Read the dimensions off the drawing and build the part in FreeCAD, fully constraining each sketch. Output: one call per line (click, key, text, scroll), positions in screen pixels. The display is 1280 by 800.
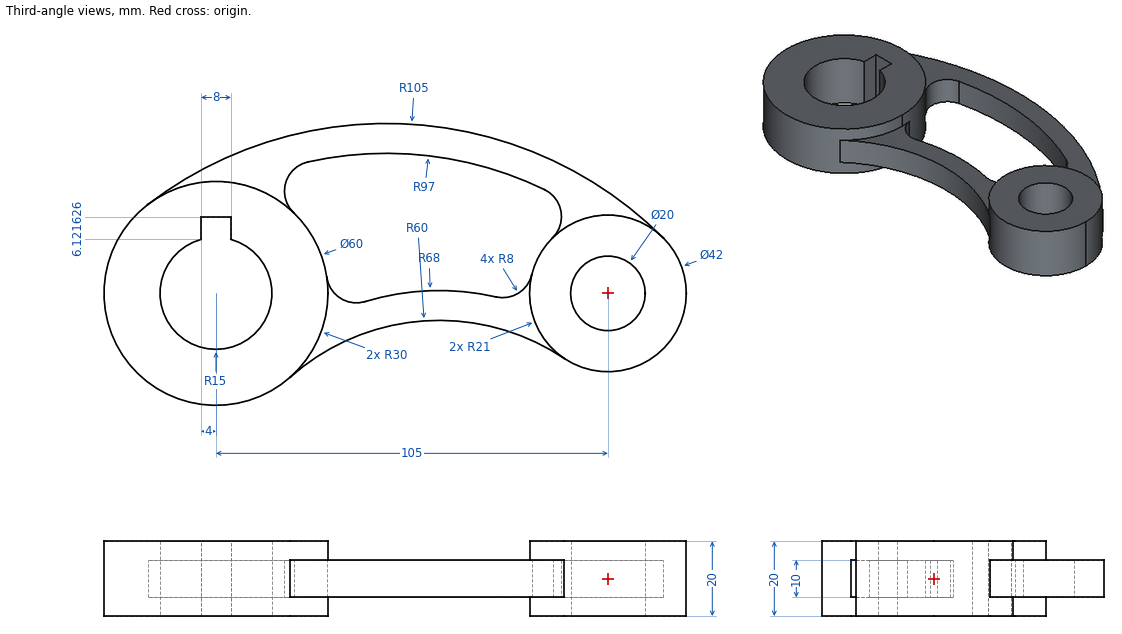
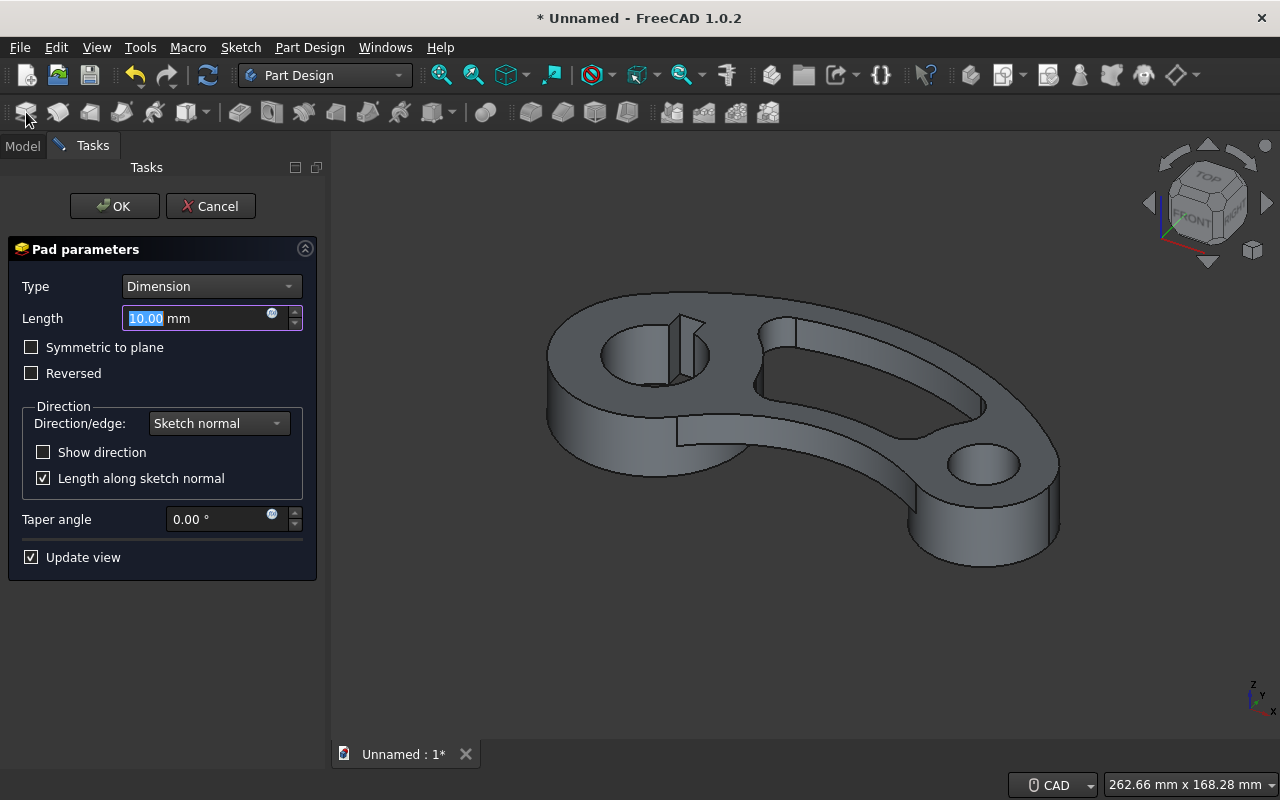
text(10)
key(Tab)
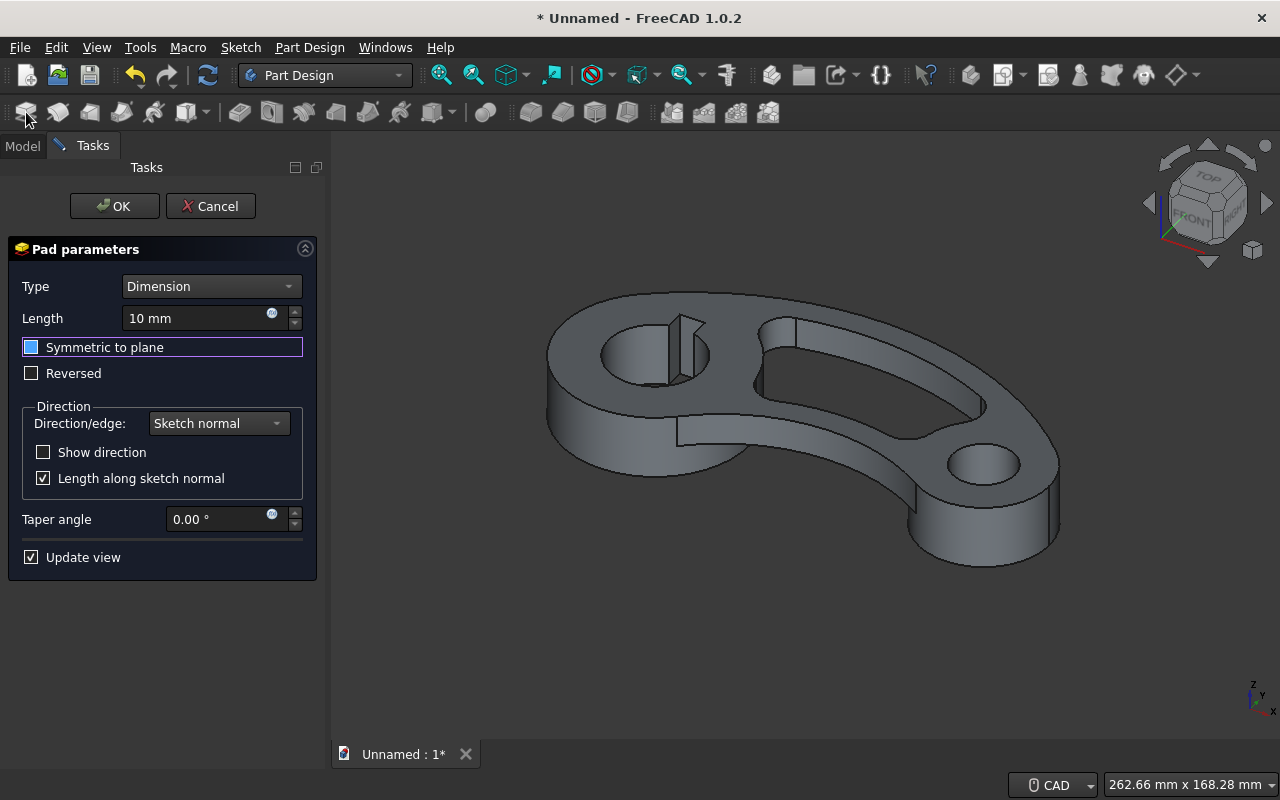
click(30, 347)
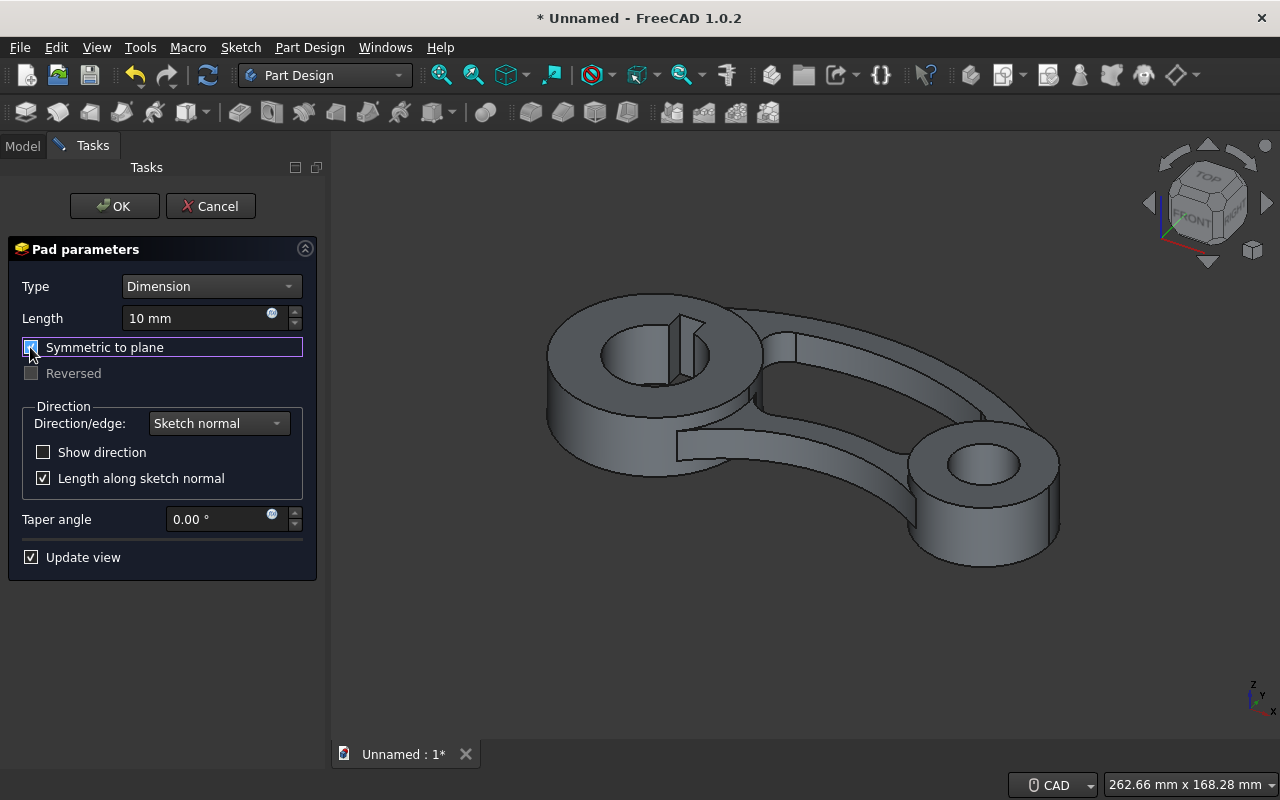
click(115, 206)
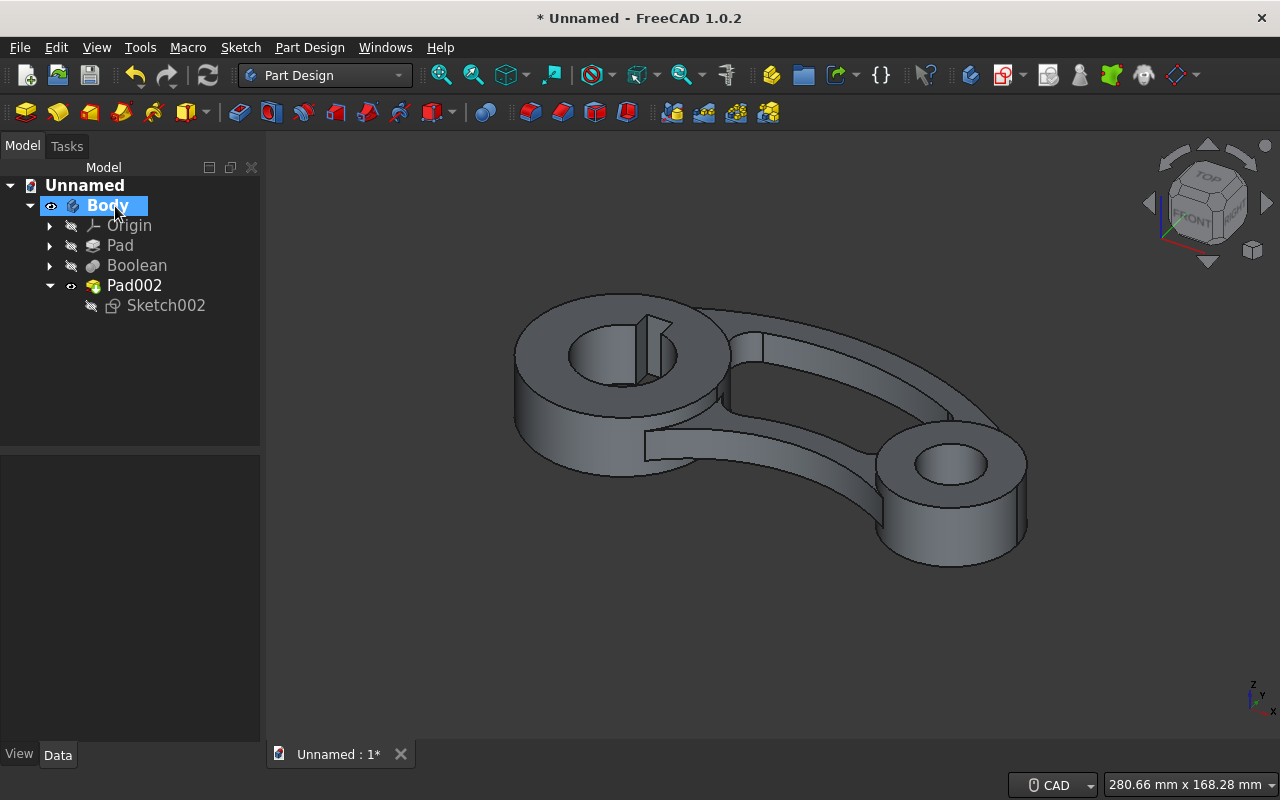
key(0)